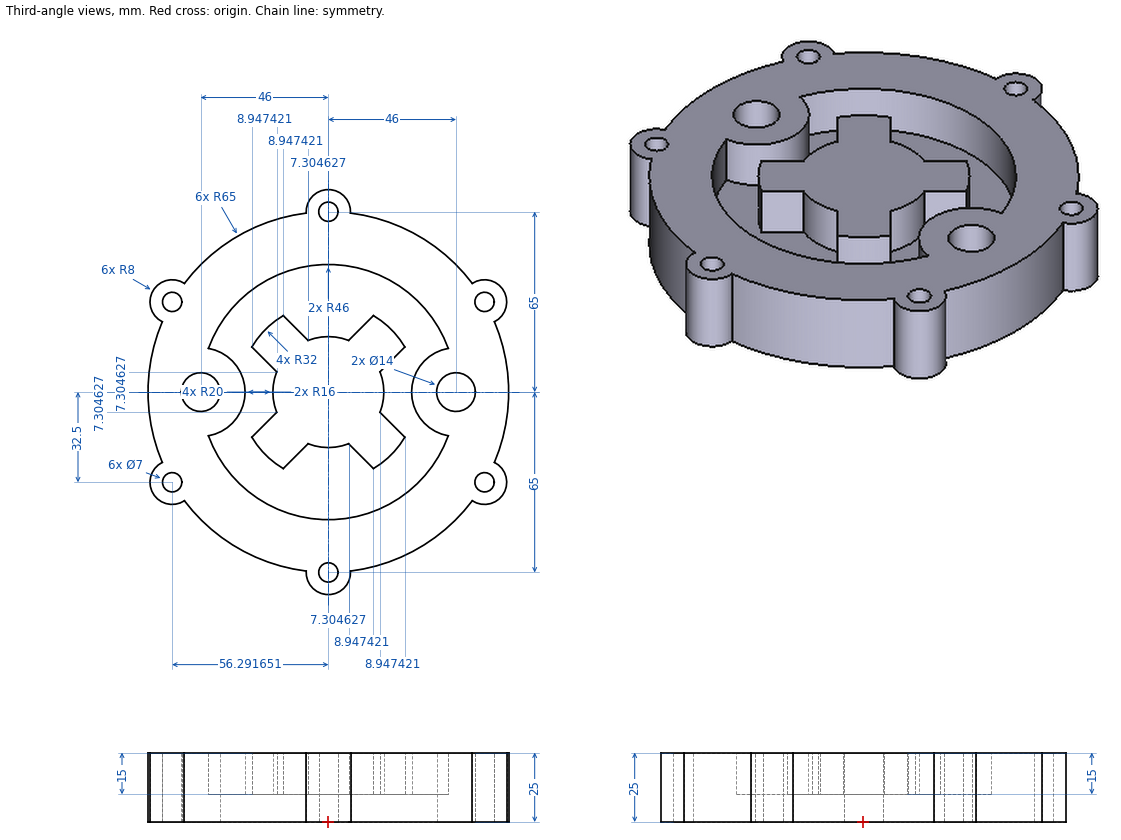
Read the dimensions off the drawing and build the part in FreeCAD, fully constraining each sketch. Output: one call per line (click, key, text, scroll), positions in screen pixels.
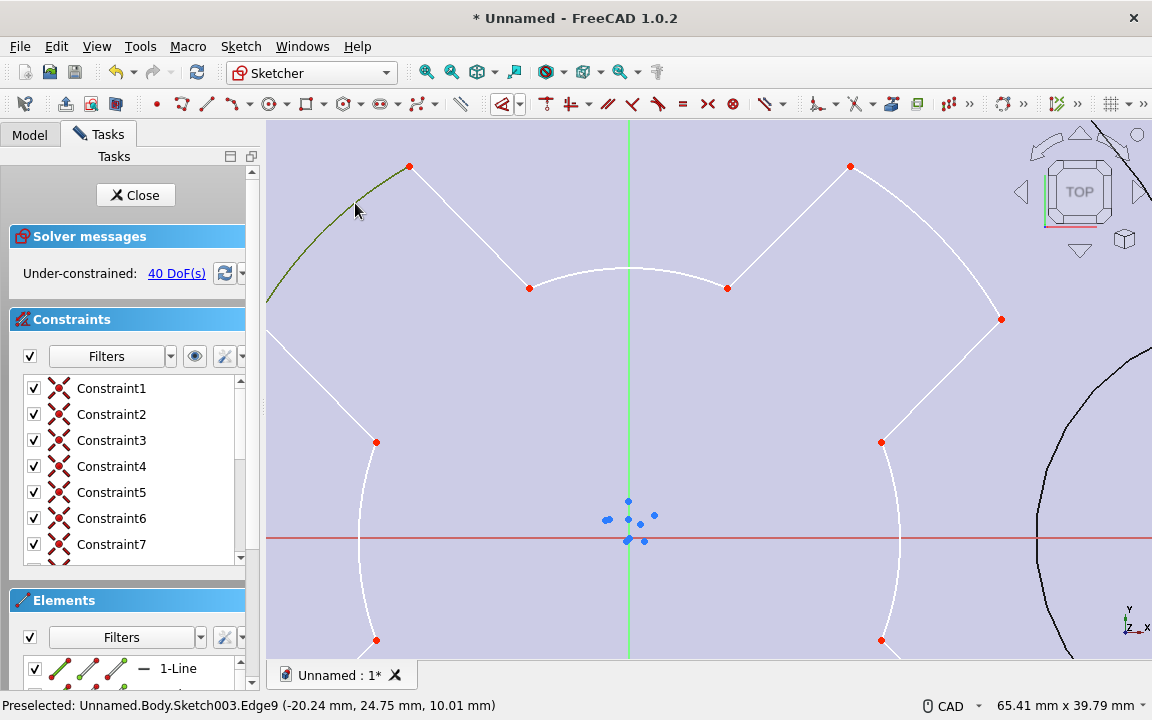
click(361, 501)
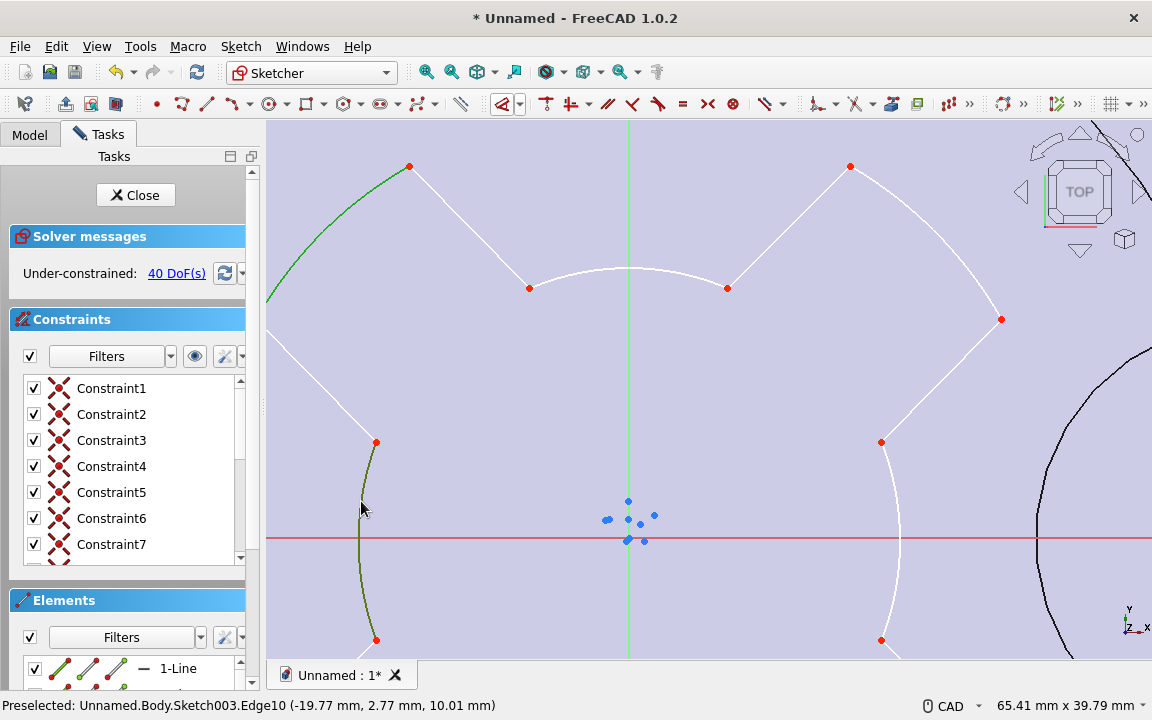
click(546, 104)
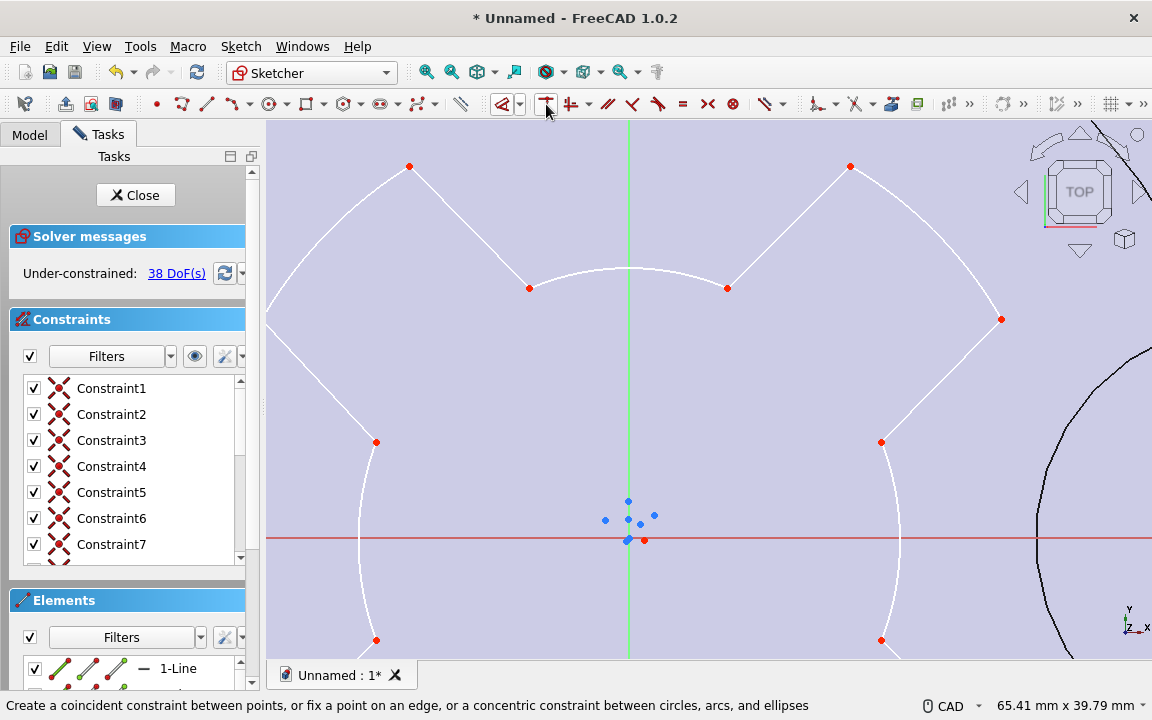
click(358, 204)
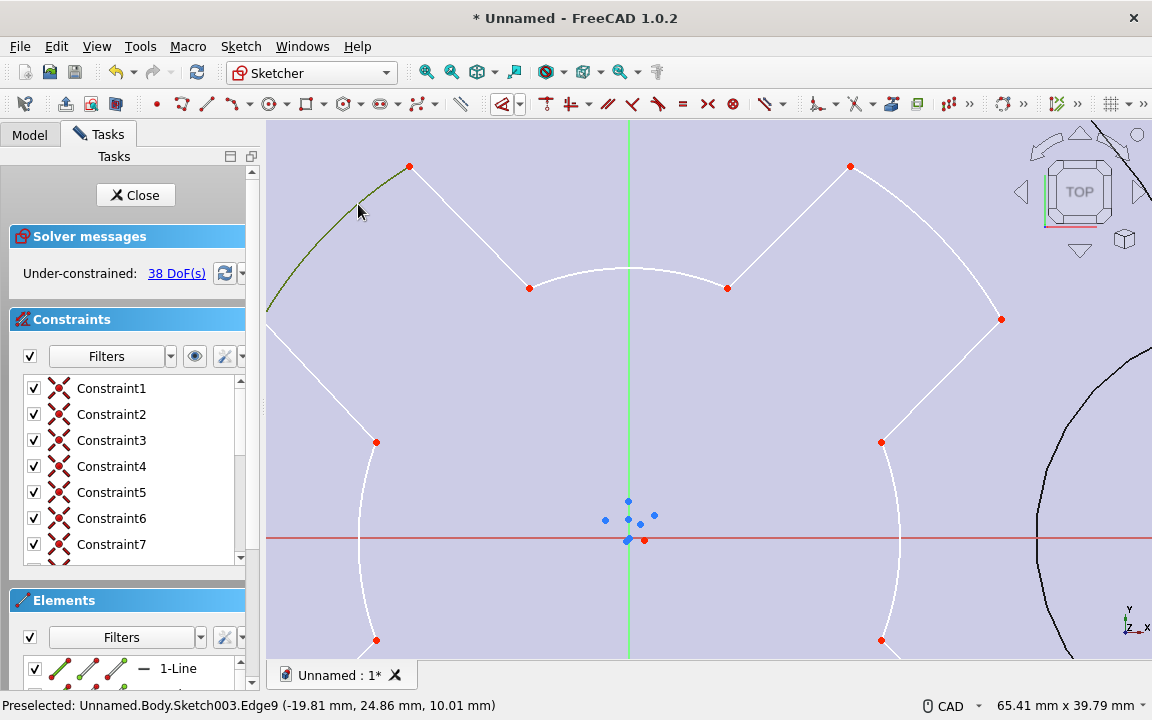
scroll(650, 268, down, 4)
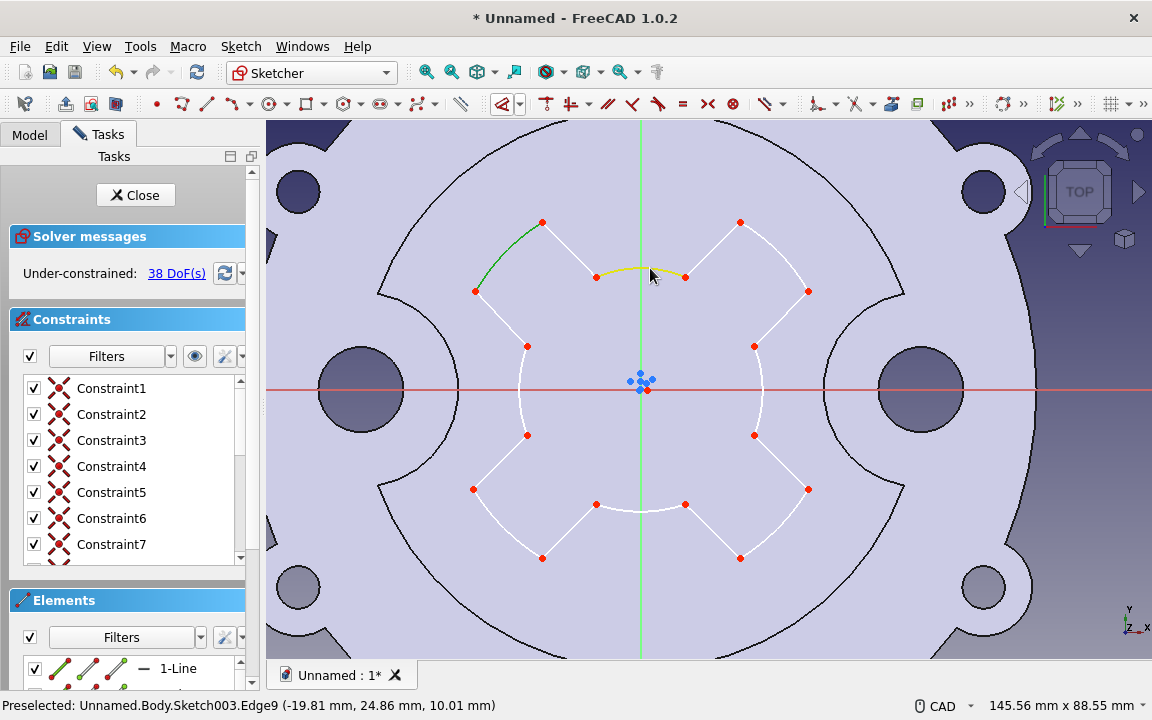
click(490, 513)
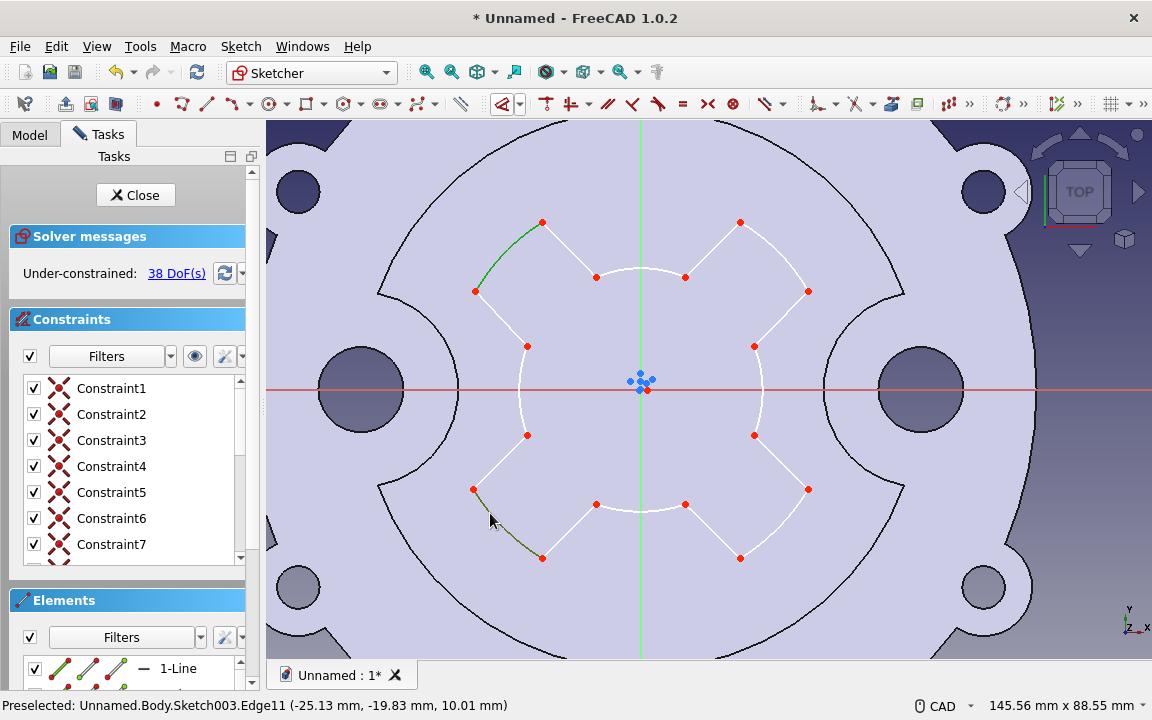
click(546, 104)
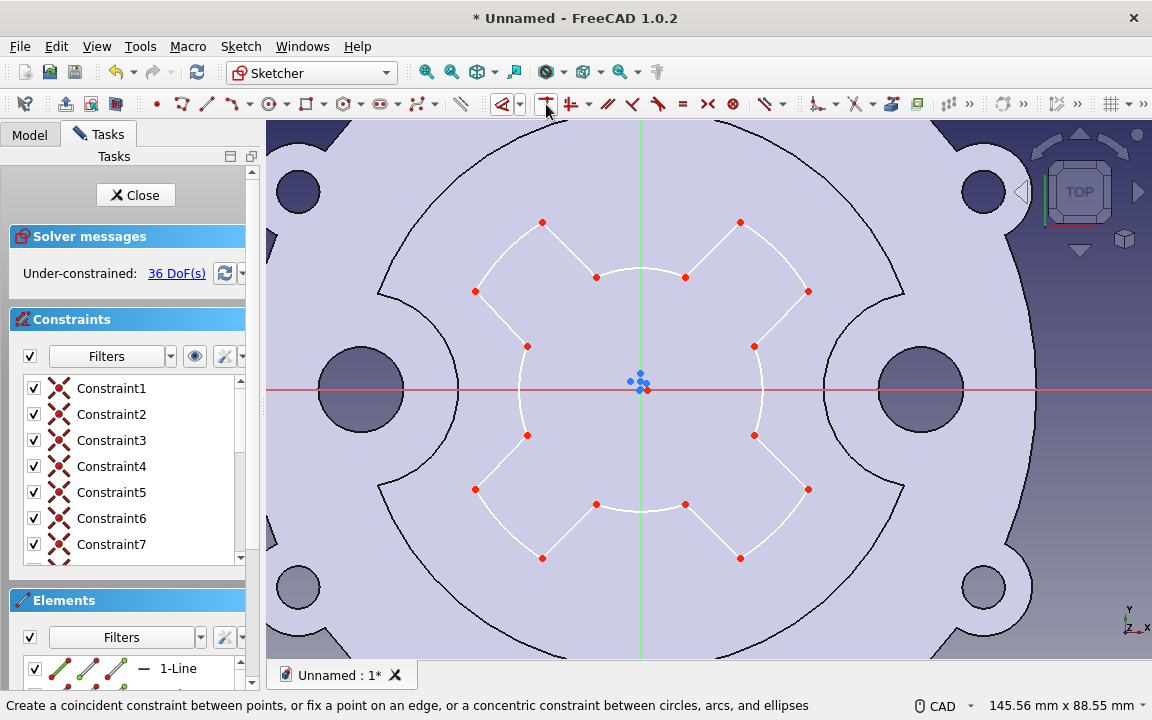
click(519, 240)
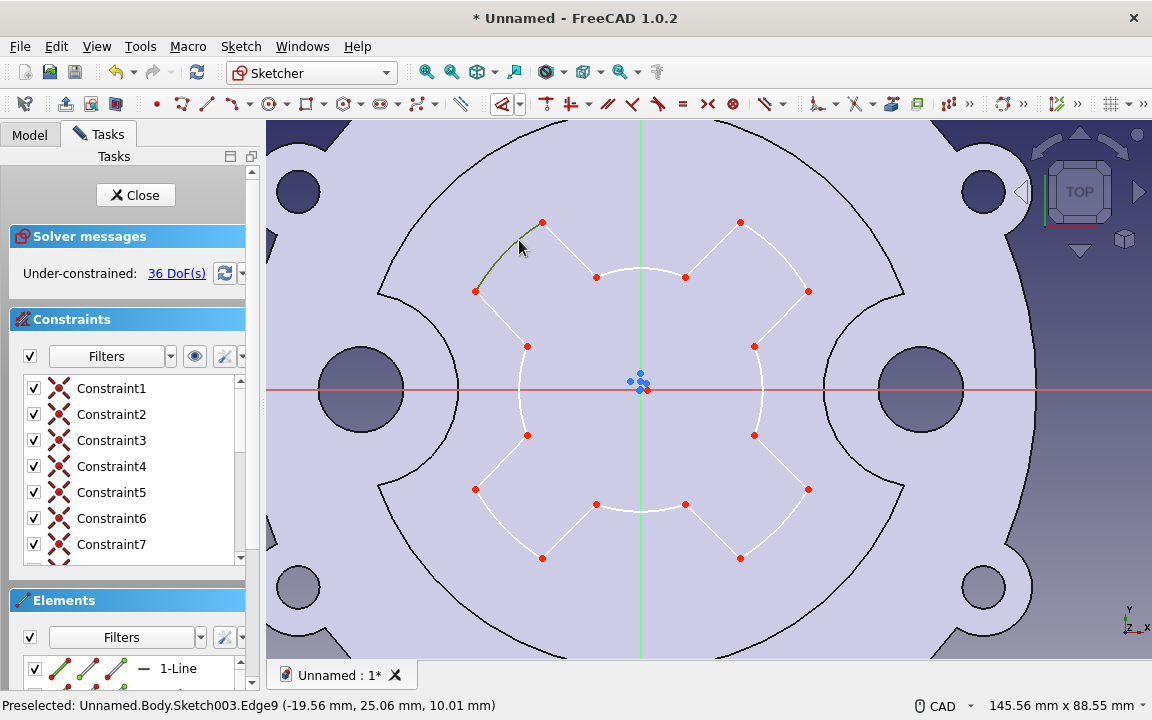
click(623, 511)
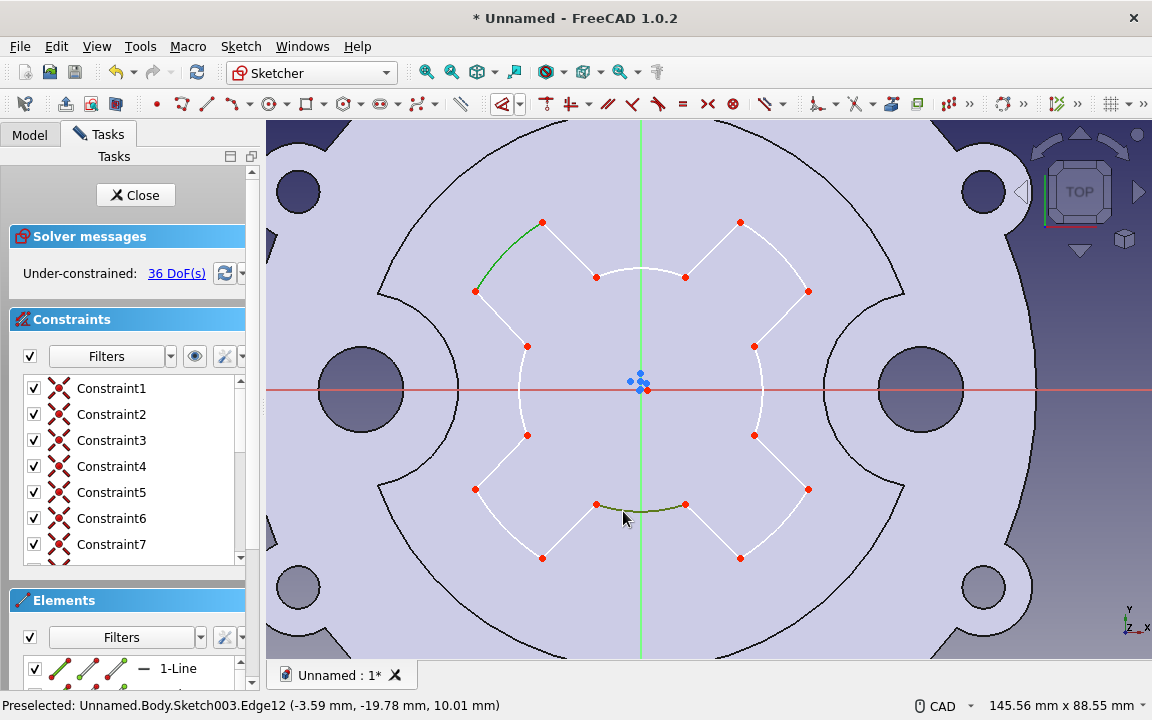
click(546, 104)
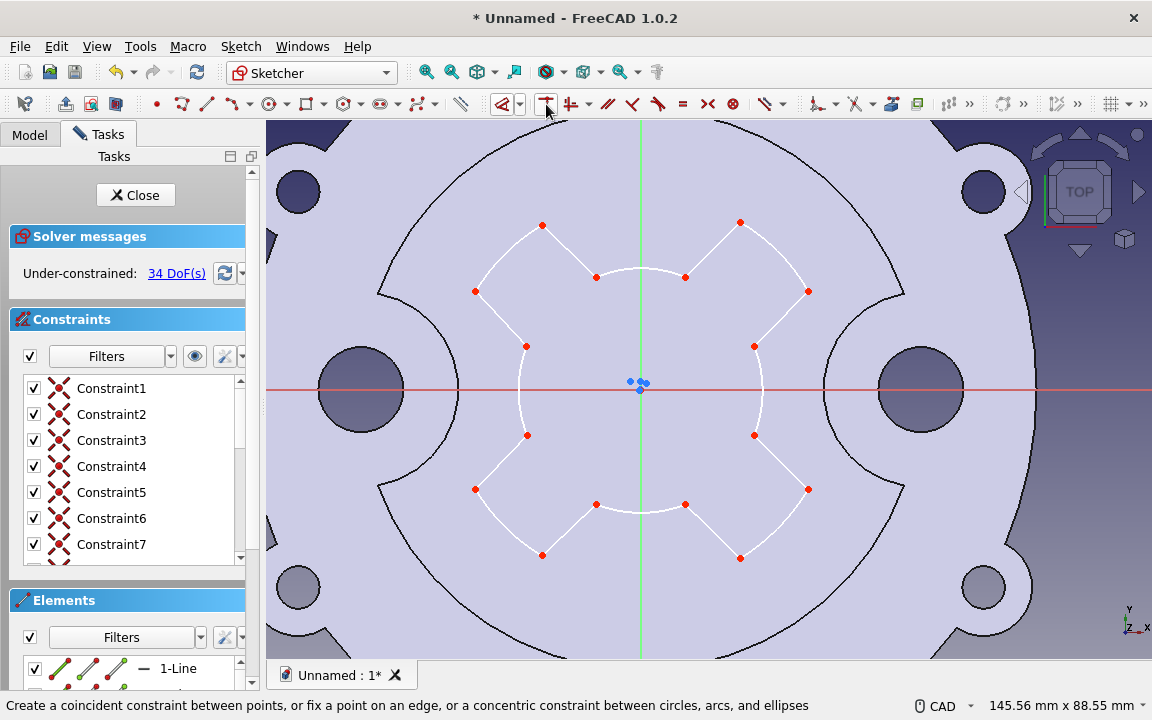
click(519, 241)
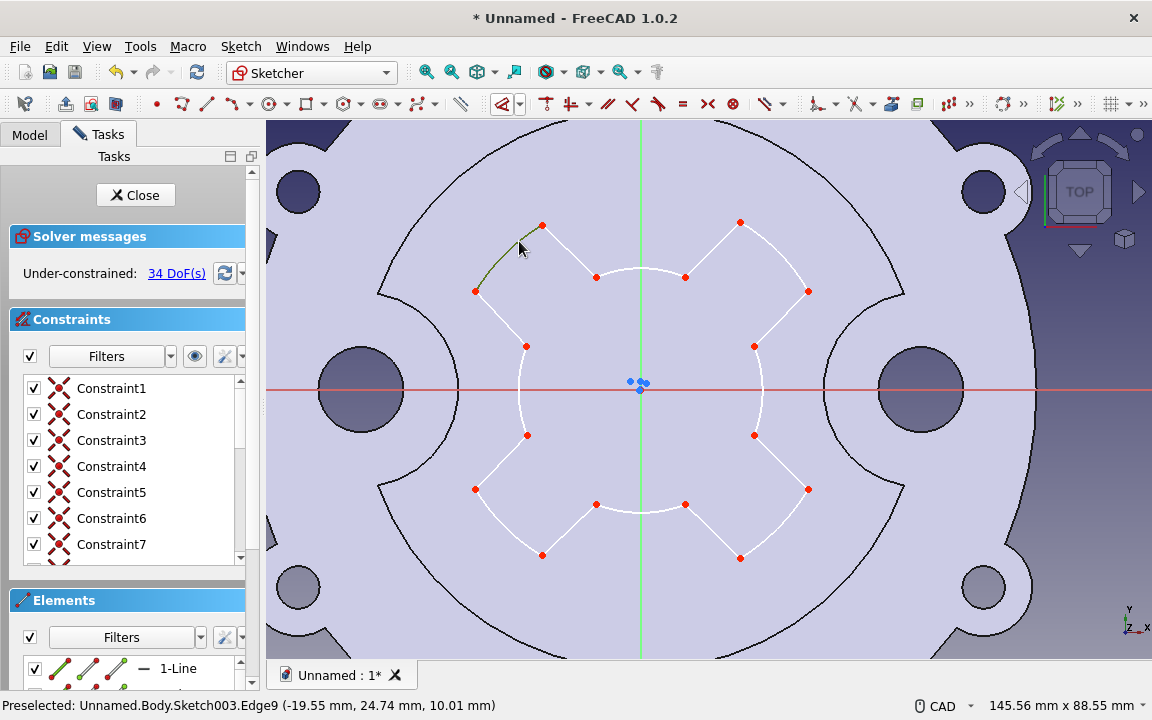
click(764, 541)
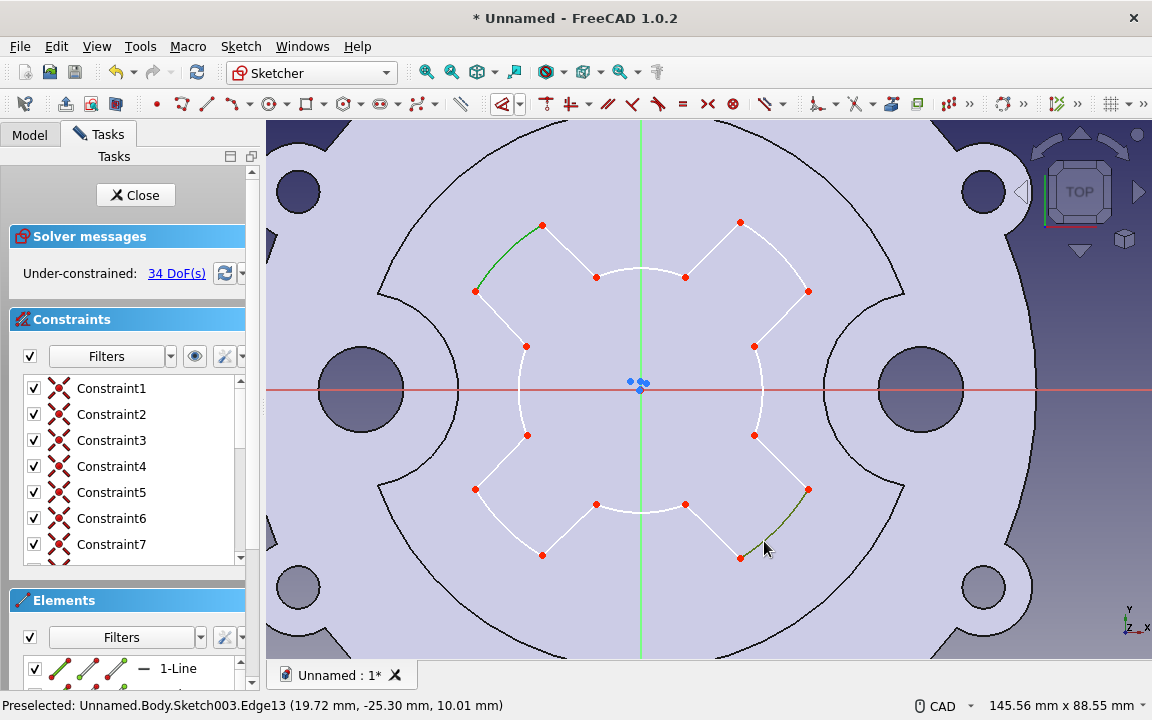
click(546, 104)